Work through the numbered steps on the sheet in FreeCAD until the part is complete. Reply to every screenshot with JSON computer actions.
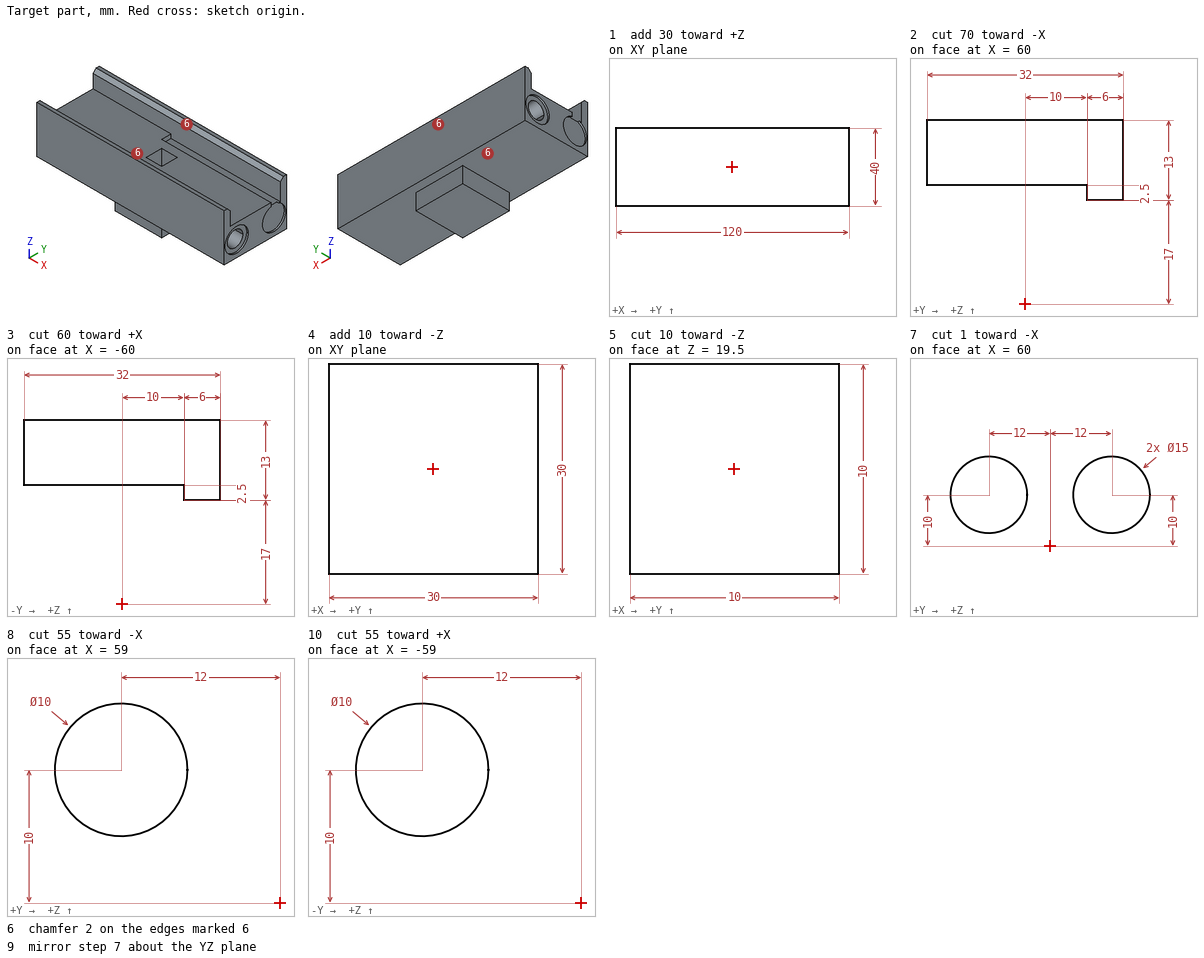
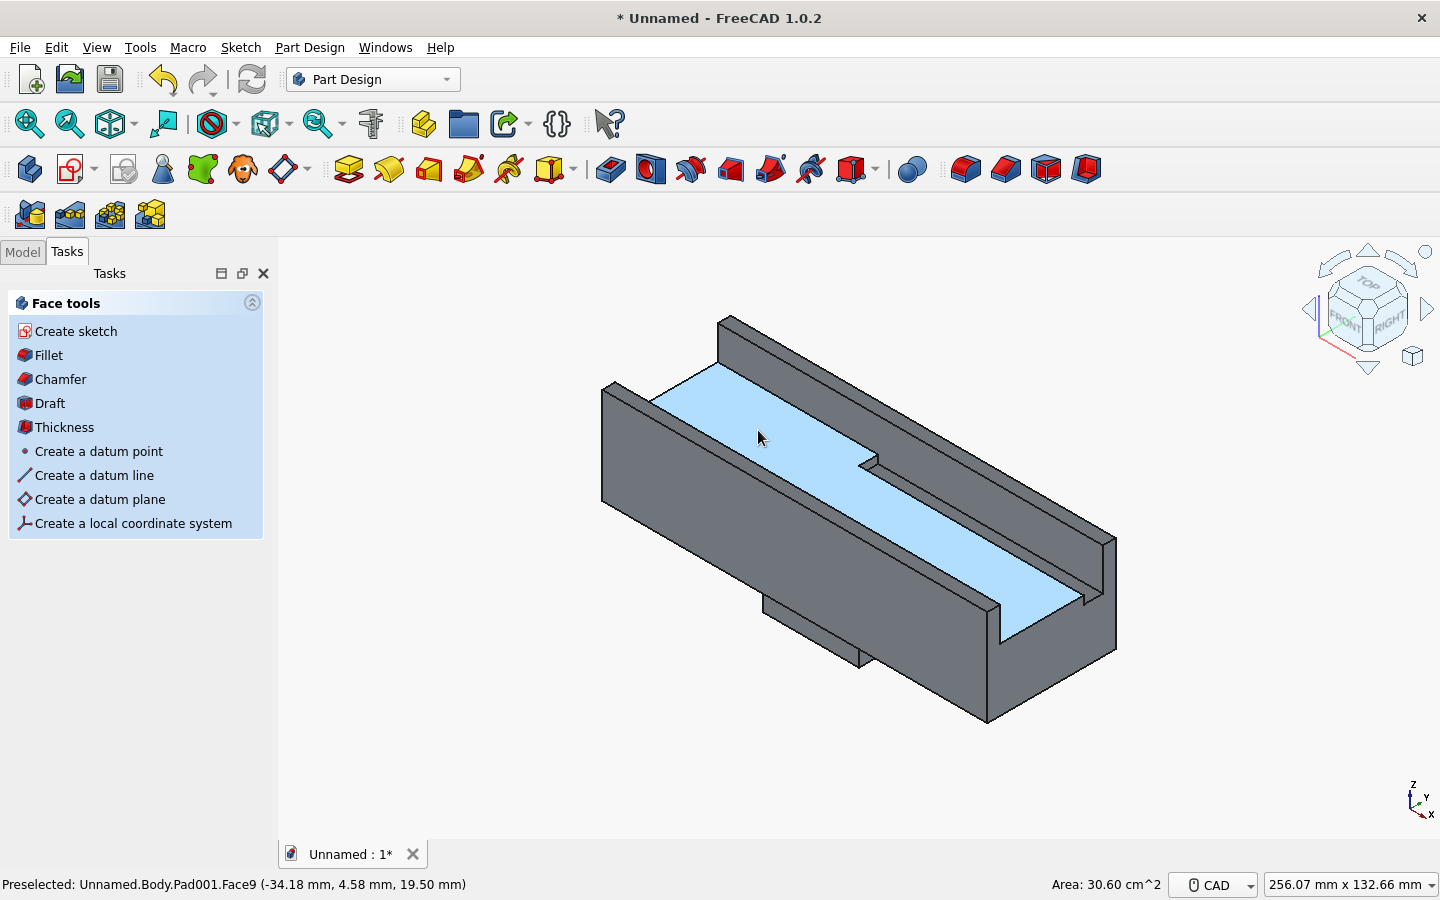
{"action": "left_click", "coordinate": [70, 170]}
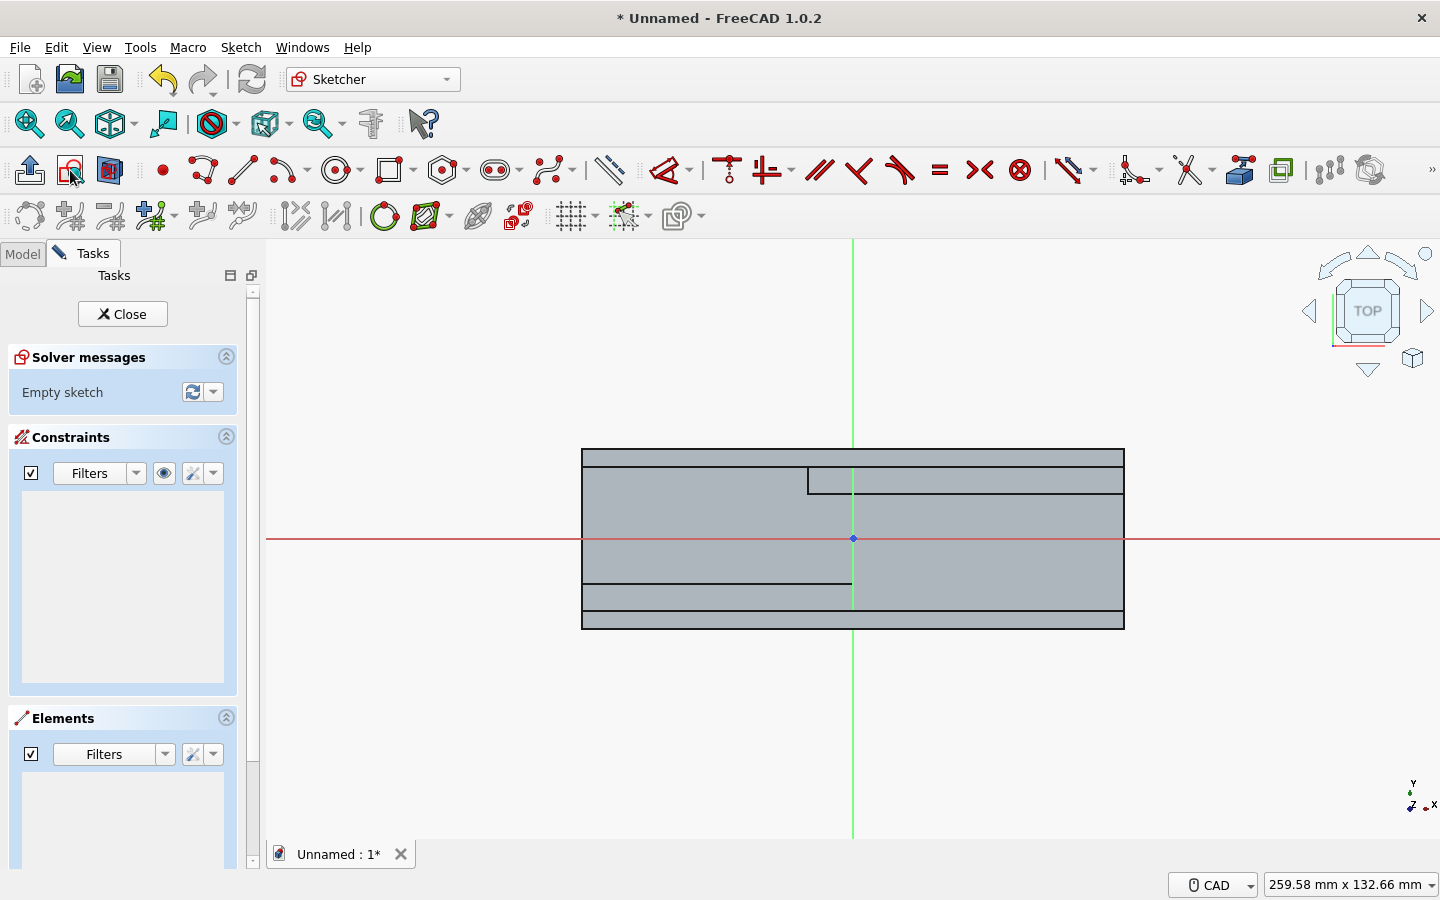
{"action": "key", "text": "q s"}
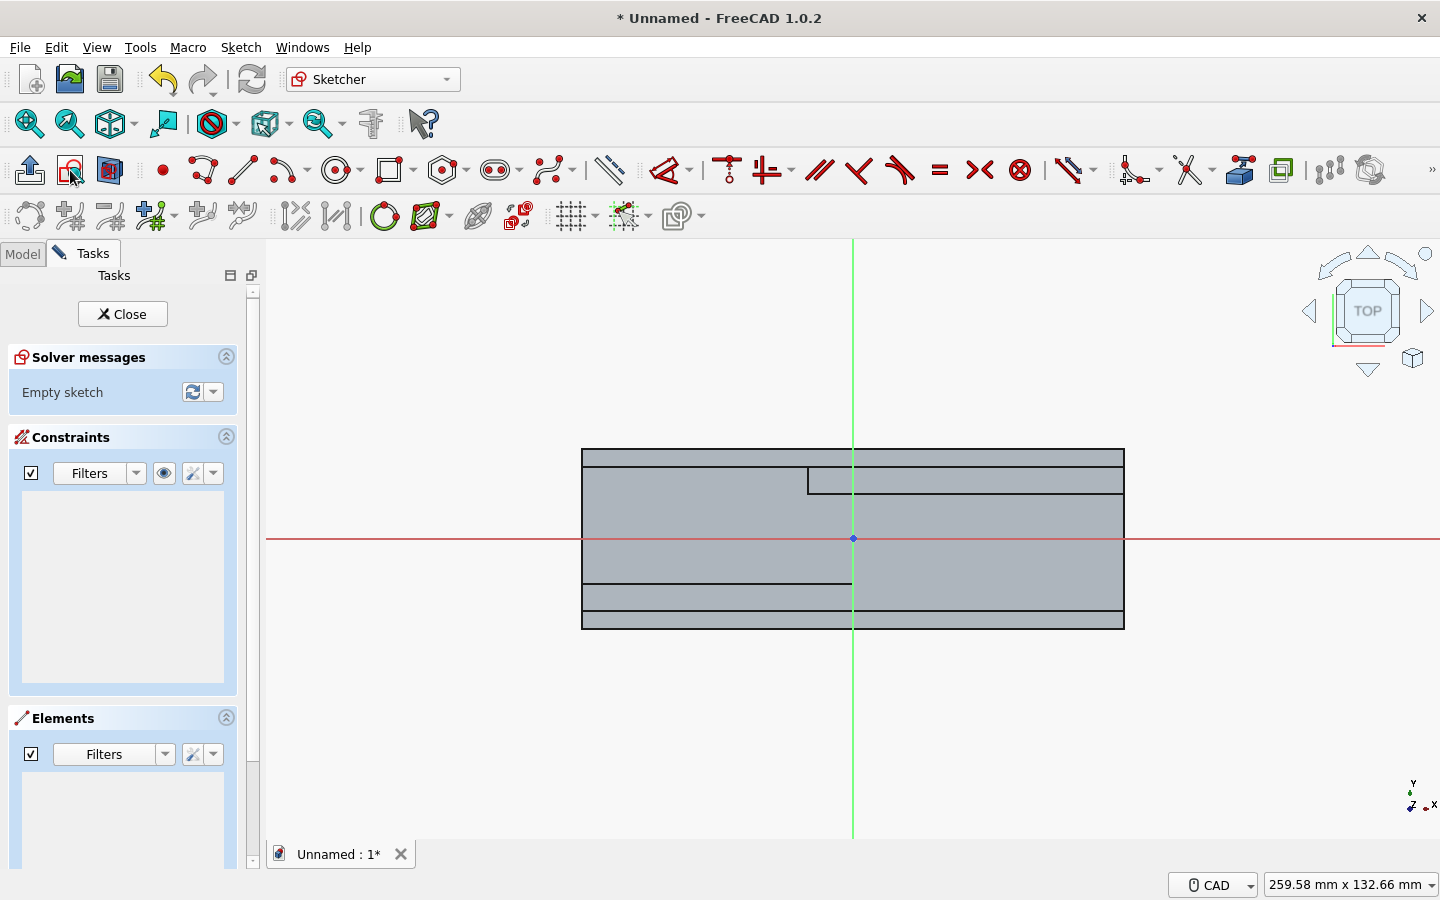
{"action": "scroll", "coordinate": [862, 539], "scroll_direction": "up", "scroll_amount": 11}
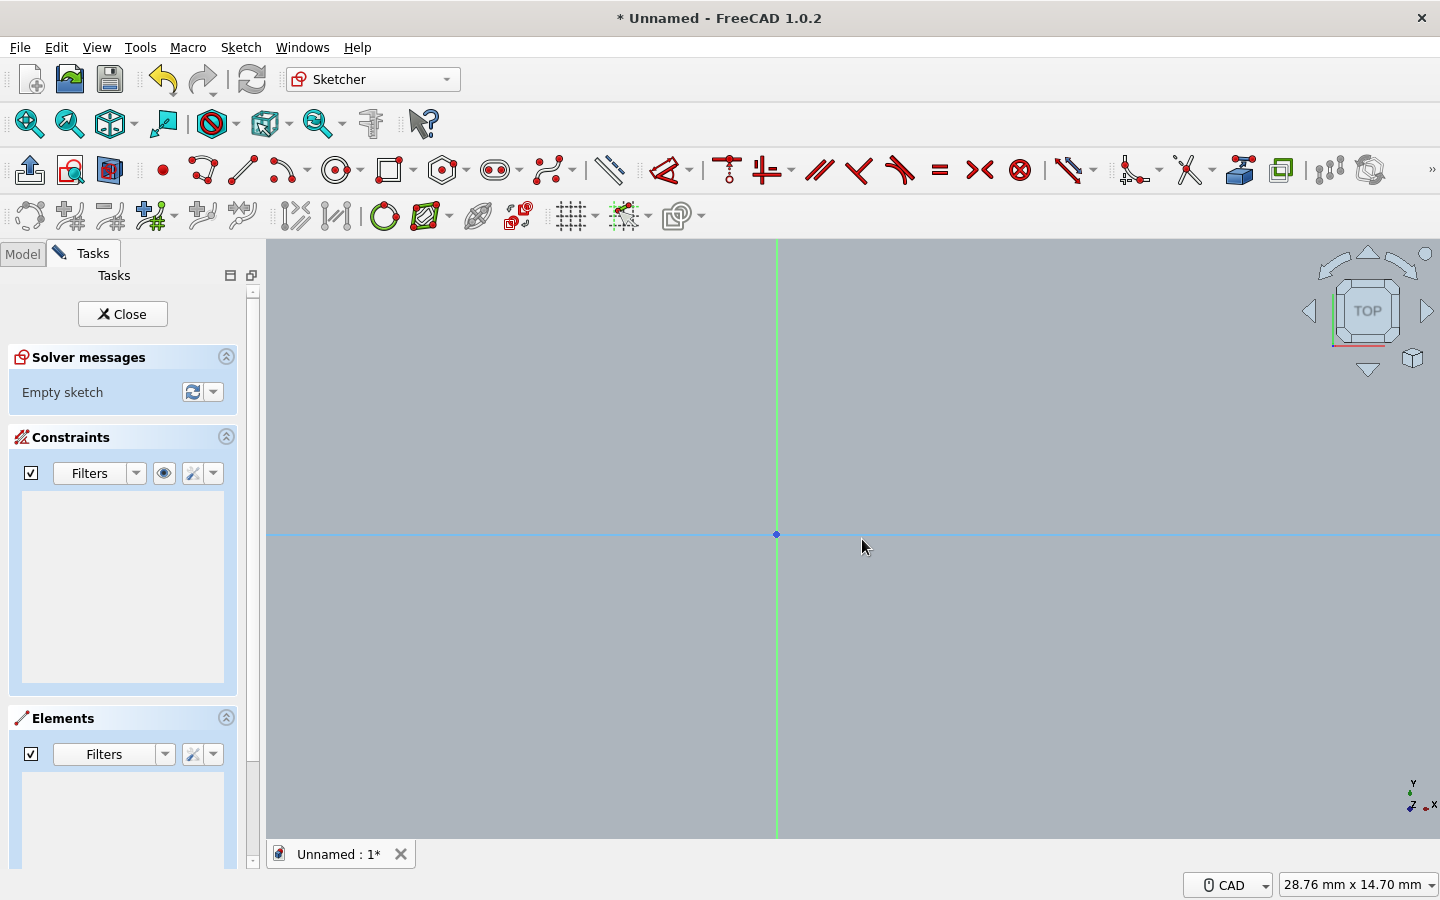
{"action": "key", "text": "g v"}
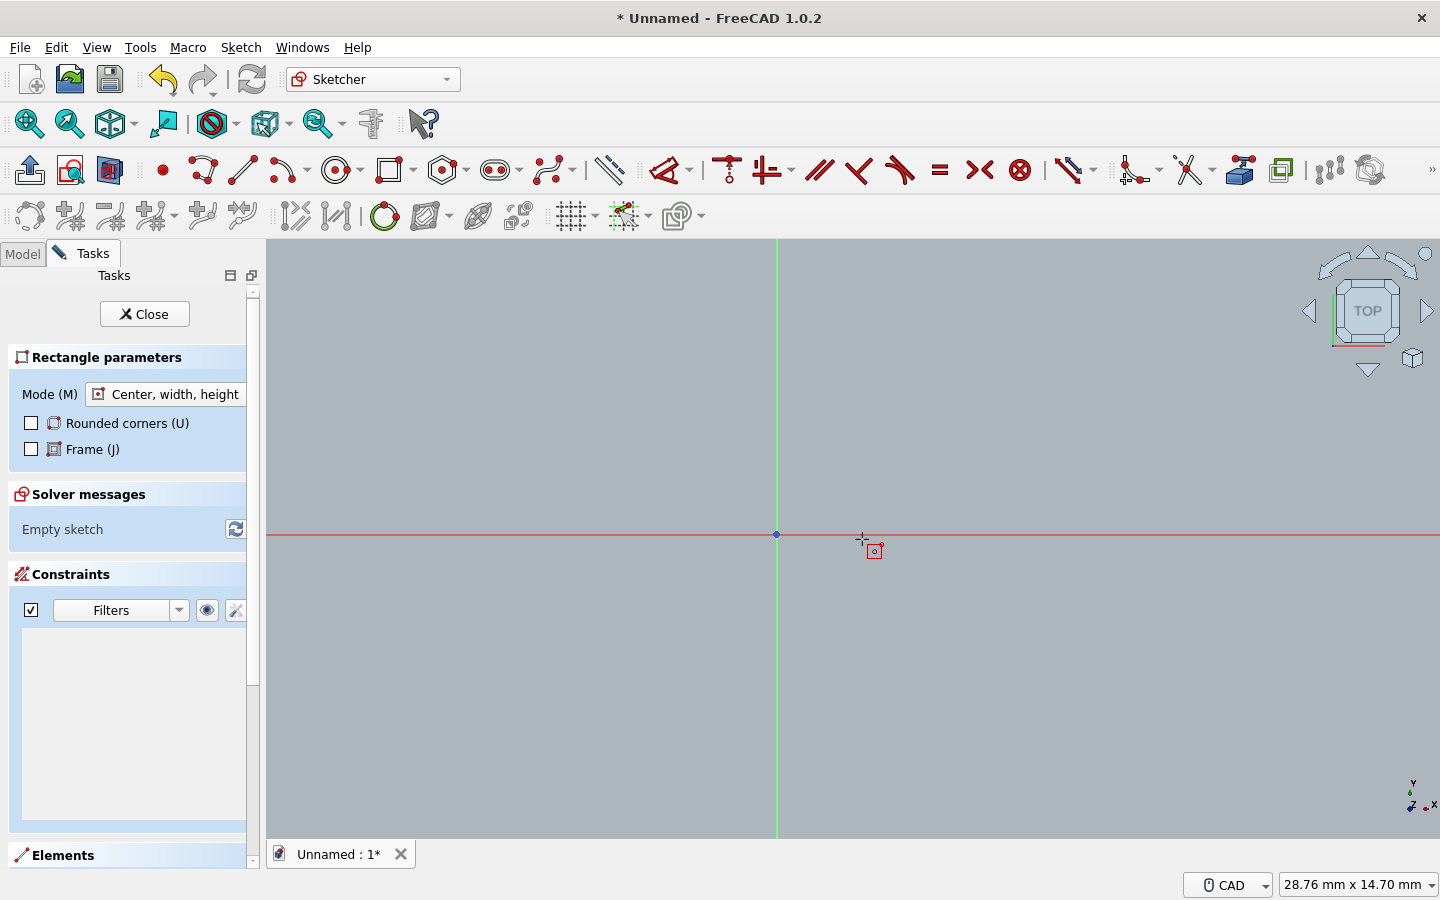
{"action": "left_click", "coordinate": [777, 535]}
{"action": "mouse_move", "coordinate": [981, 331]}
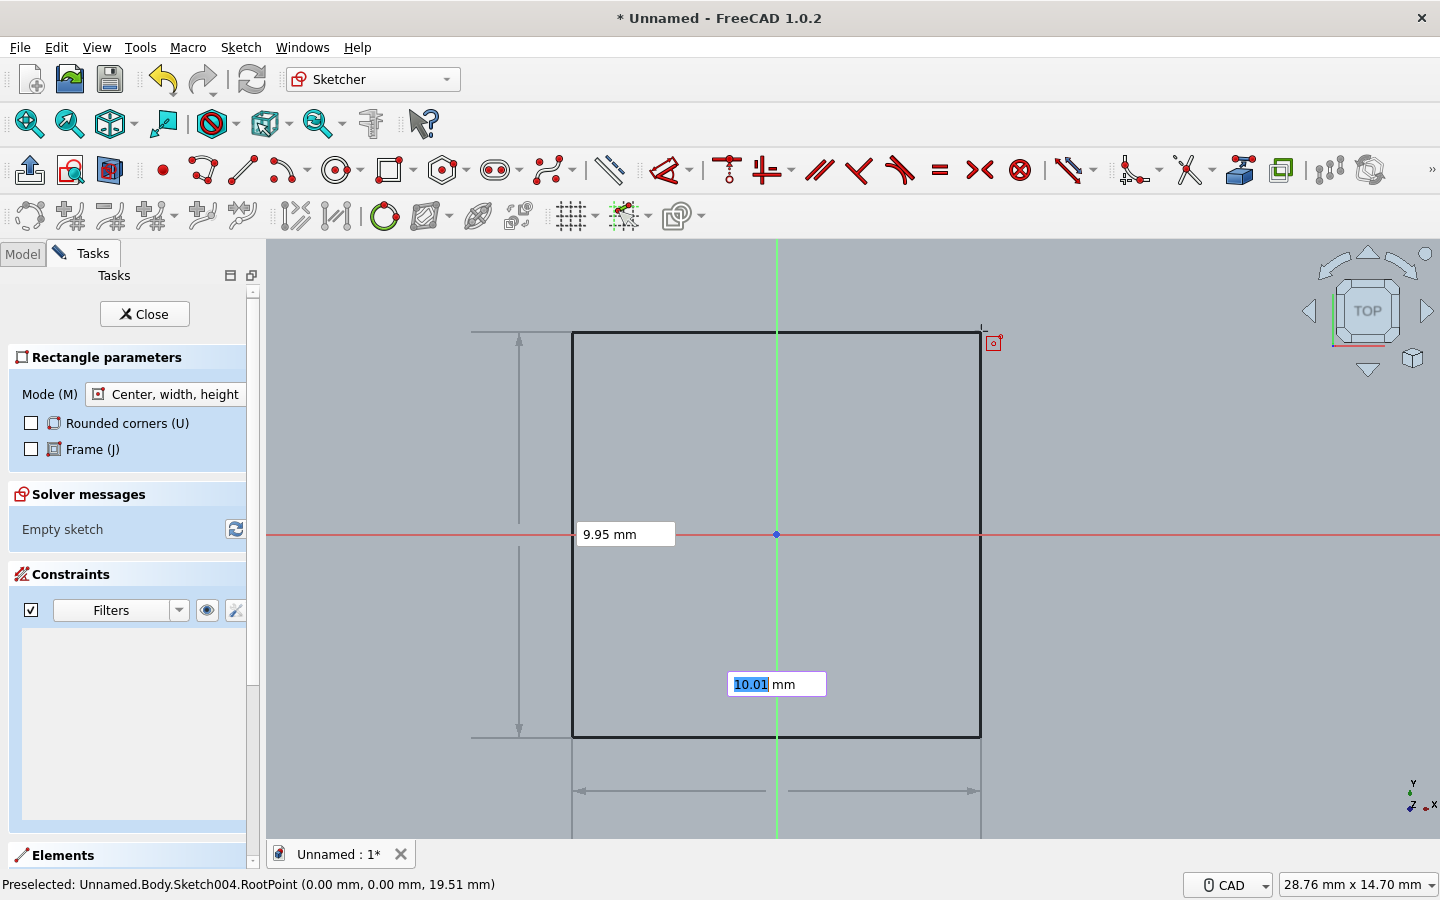
{"action": "type", "text": "10"}
{"action": "key", "text": "Tab"}
{"action": "type", "text": "10"}
{"action": "key", "text": "Return"}
{"action": "key", "text": "Escape"}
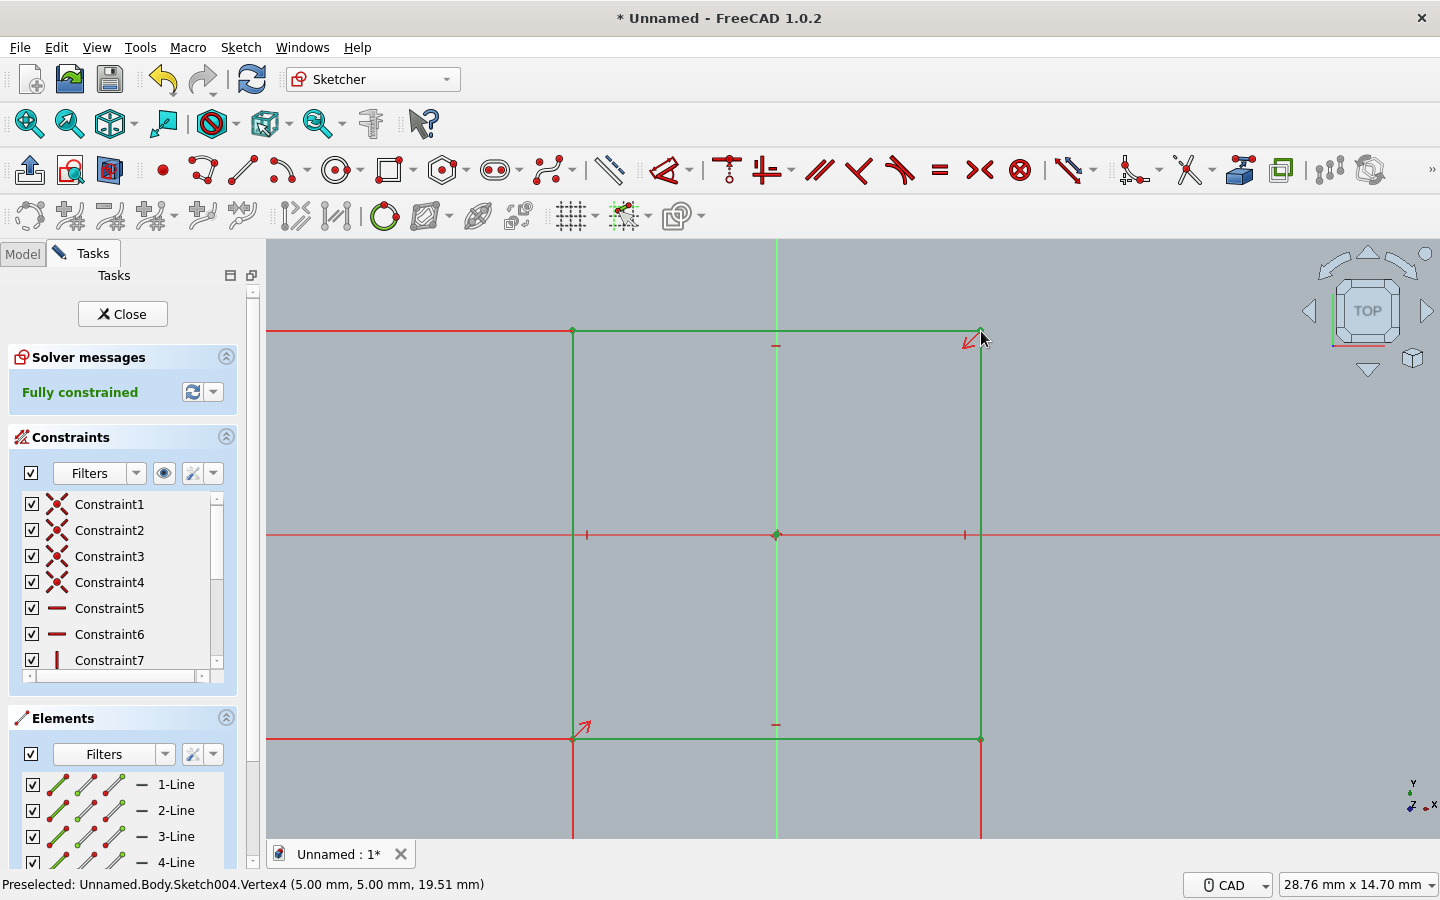
{"action": "left_click", "coordinate": [123, 314]}